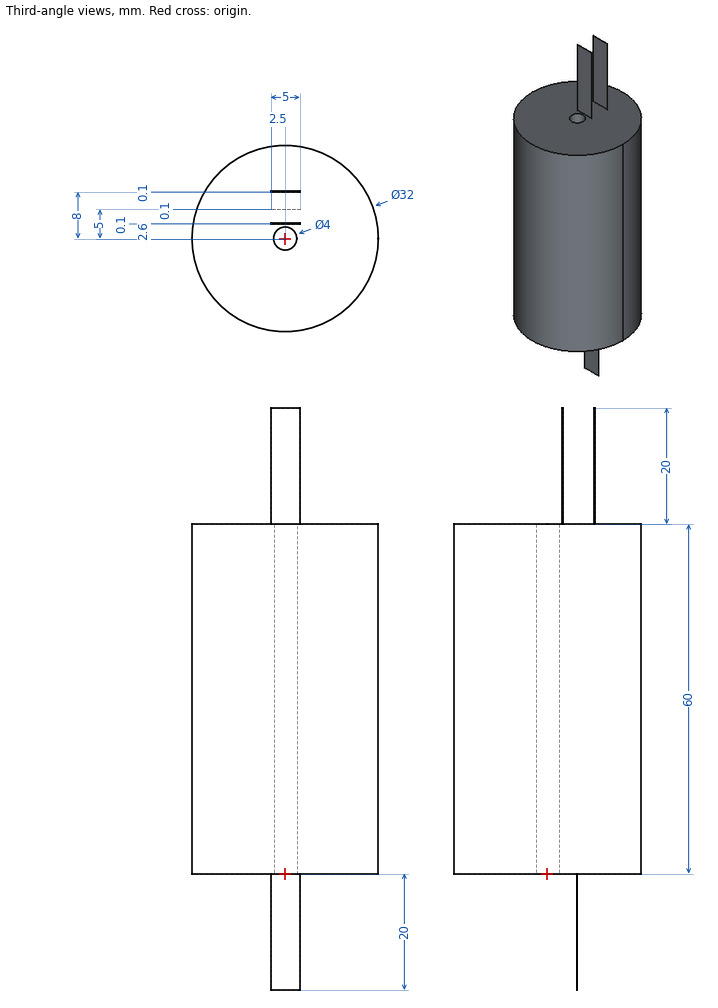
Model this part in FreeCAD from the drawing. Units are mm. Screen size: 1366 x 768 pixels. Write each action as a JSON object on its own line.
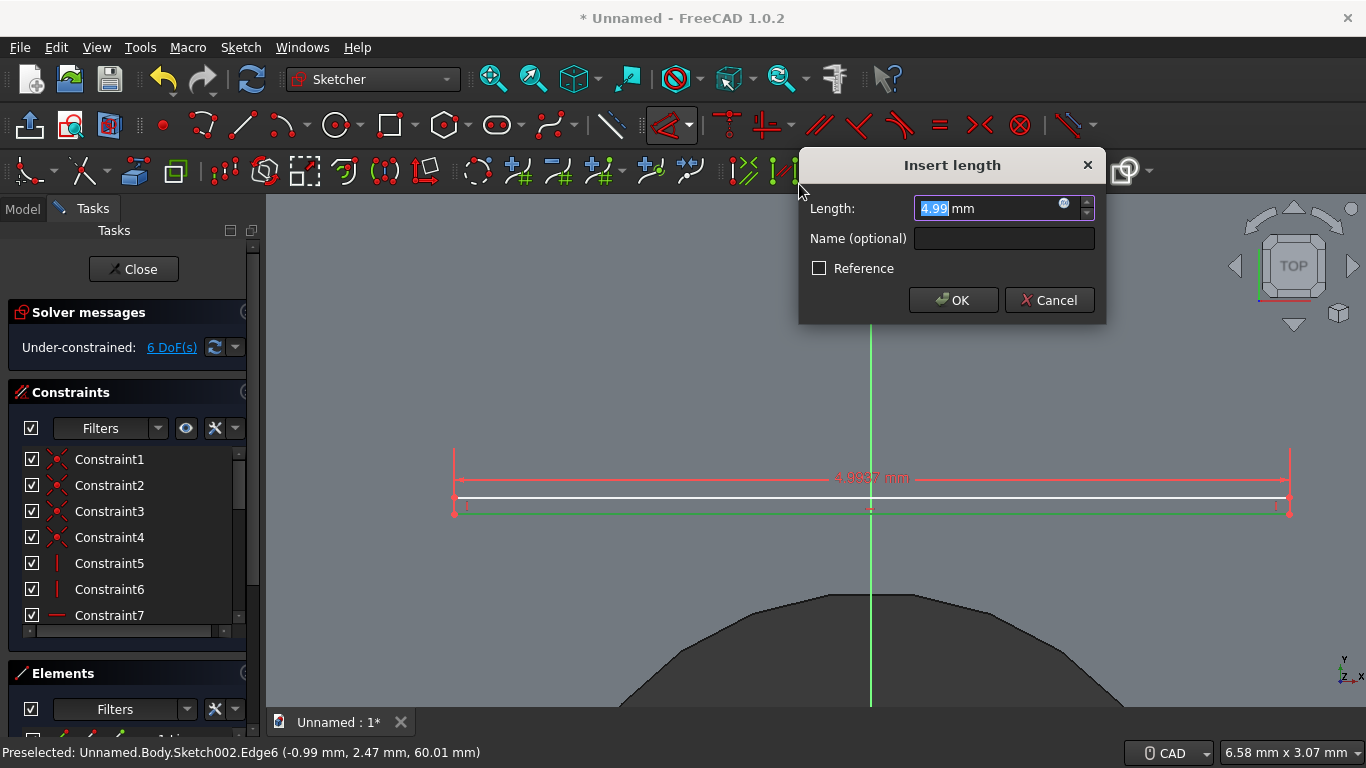
{"action": "type", "text": "5"}
{"action": "key", "text": "Return"}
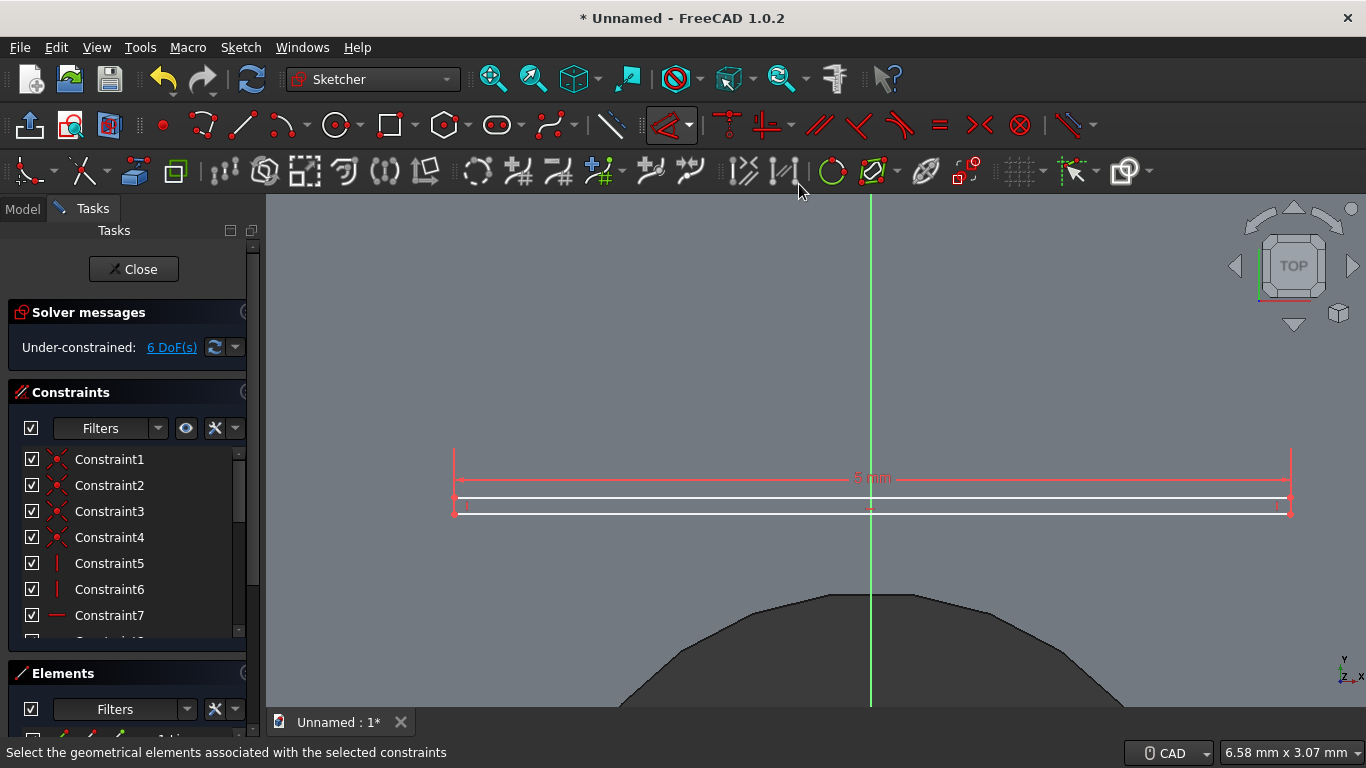
{"action": "scroll", "coordinate": [707, 516], "scroll_direction": "down", "scroll_amount": 7}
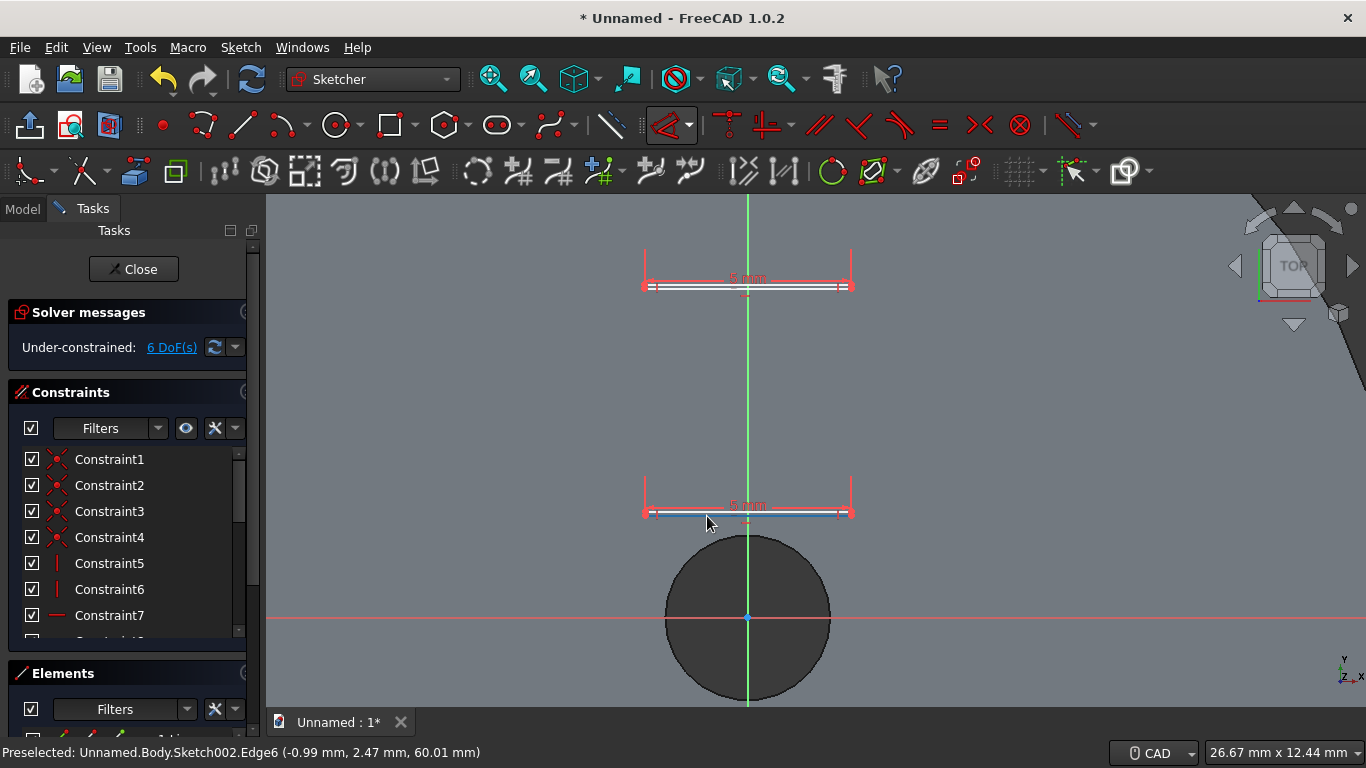
{"action": "scroll", "coordinate": [645, 289], "scroll_direction": "up", "scroll_amount": 6}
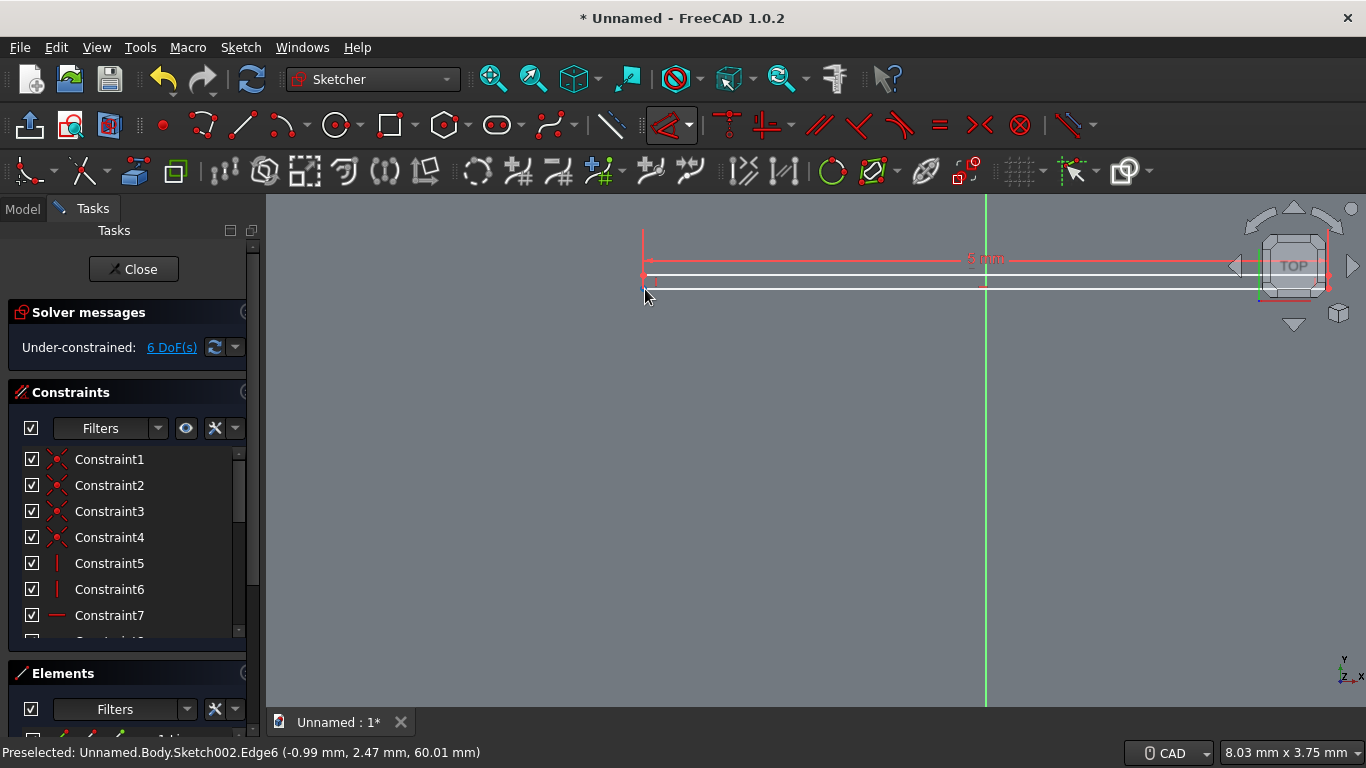
{"action": "left_click", "coordinate": [643, 289]}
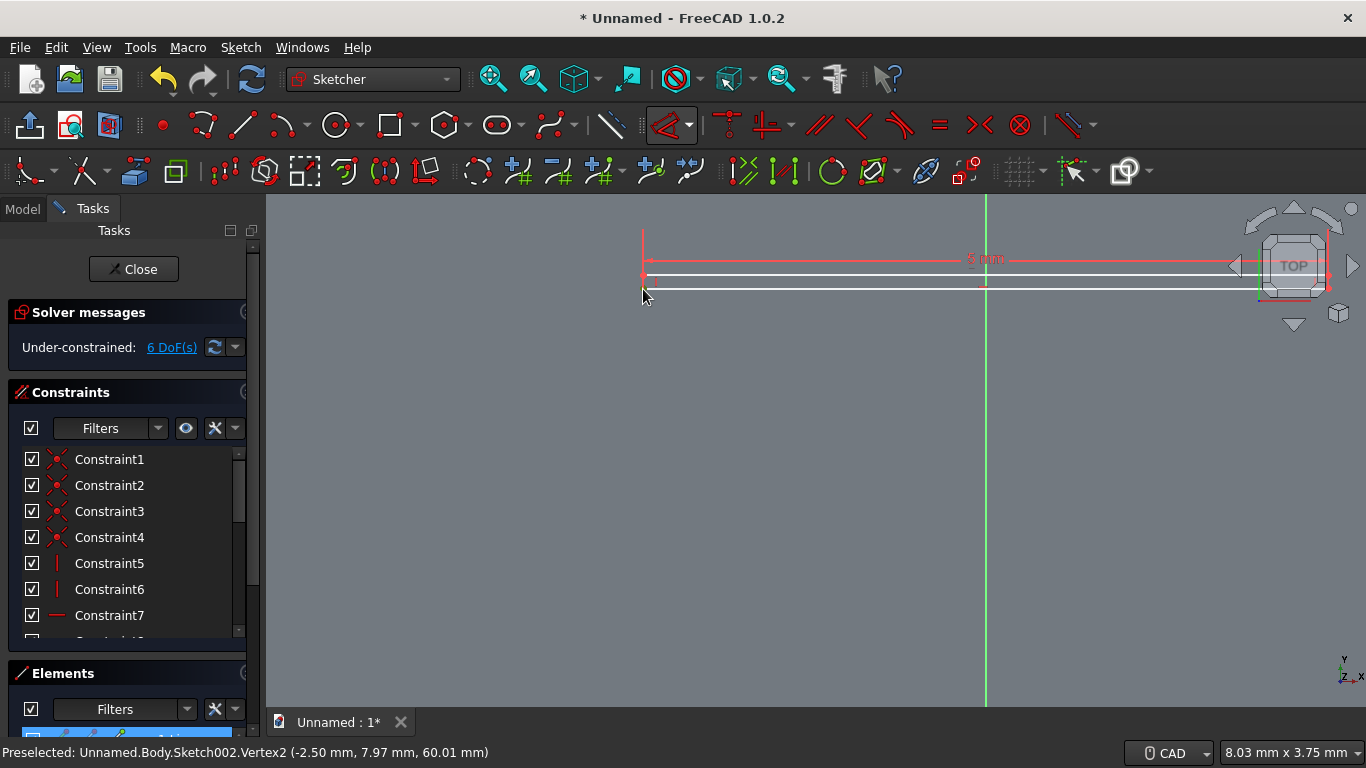
{"action": "left_click", "coordinate": [692, 126]}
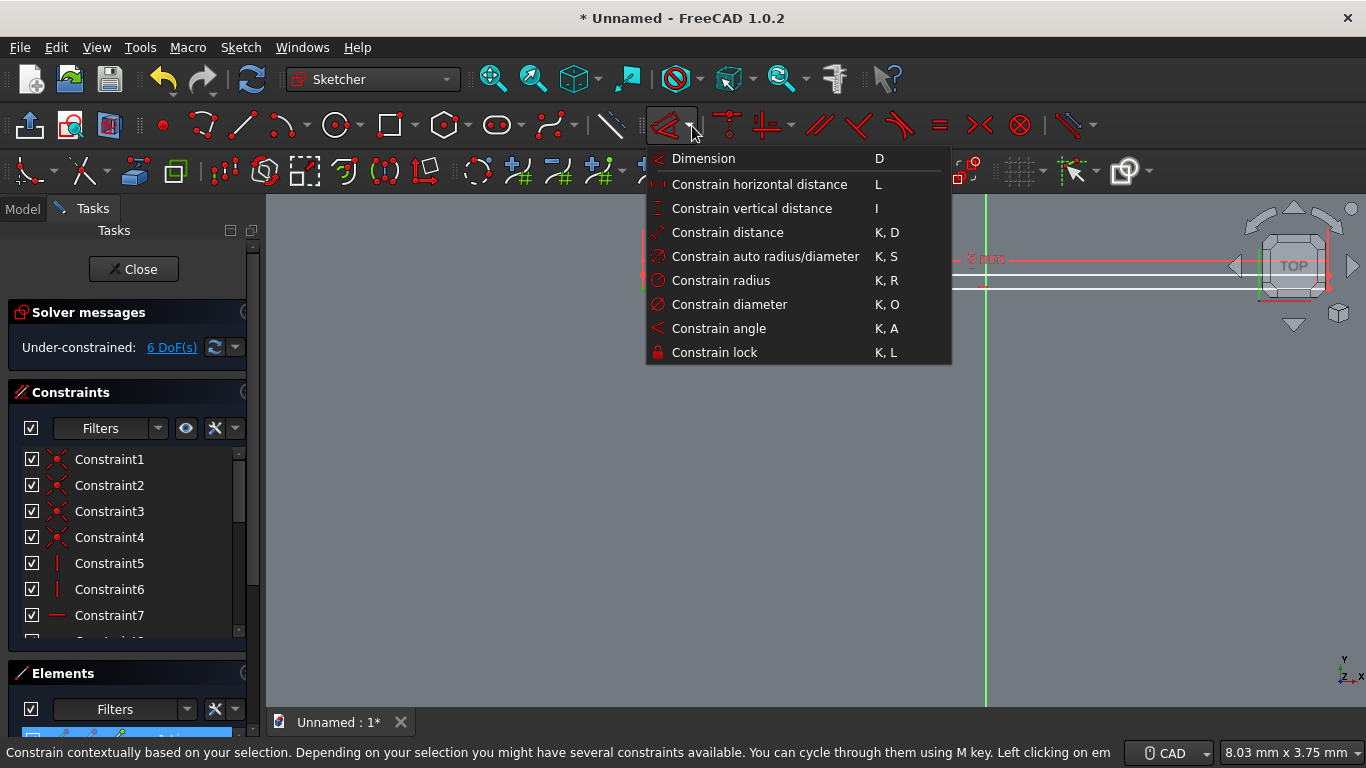
{"action": "left_click", "coordinate": [799, 208]}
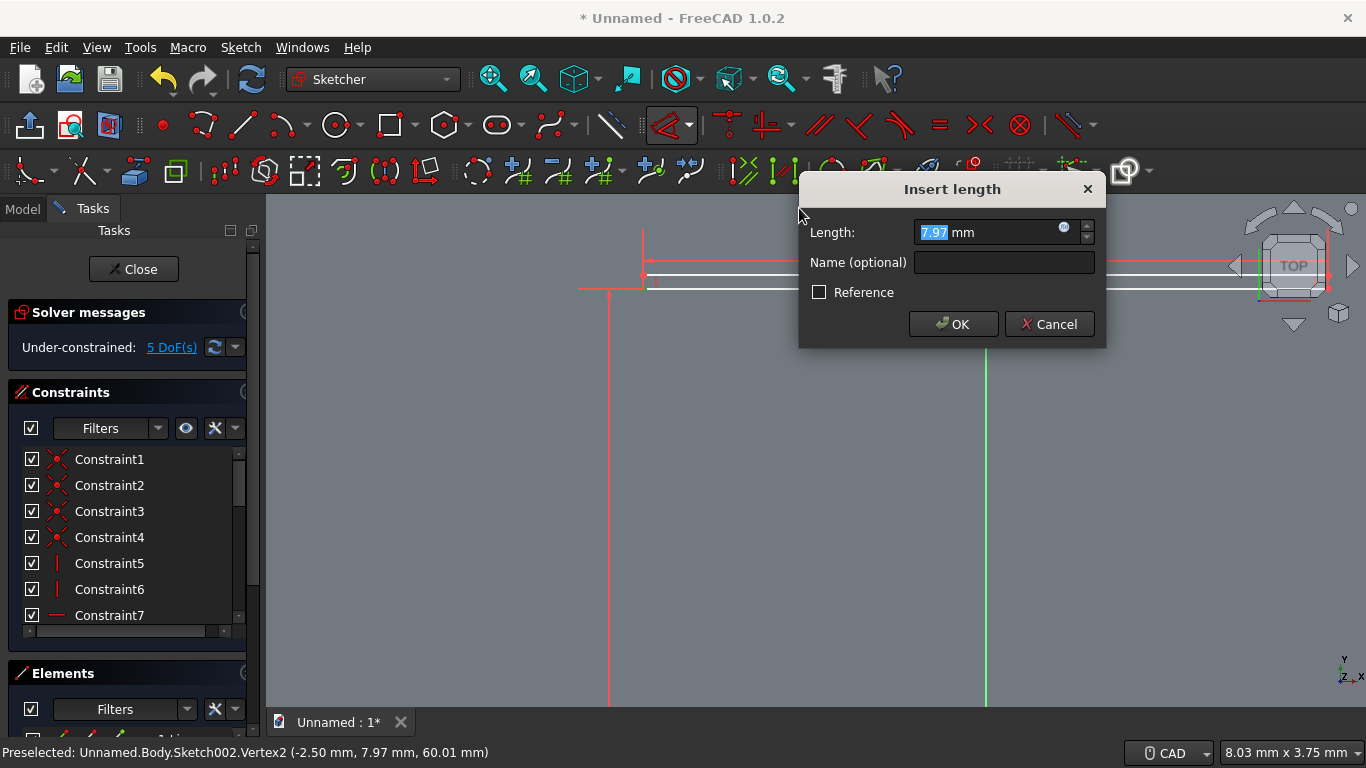
{"action": "type", "text": "8"}
{"action": "key", "text": "Return"}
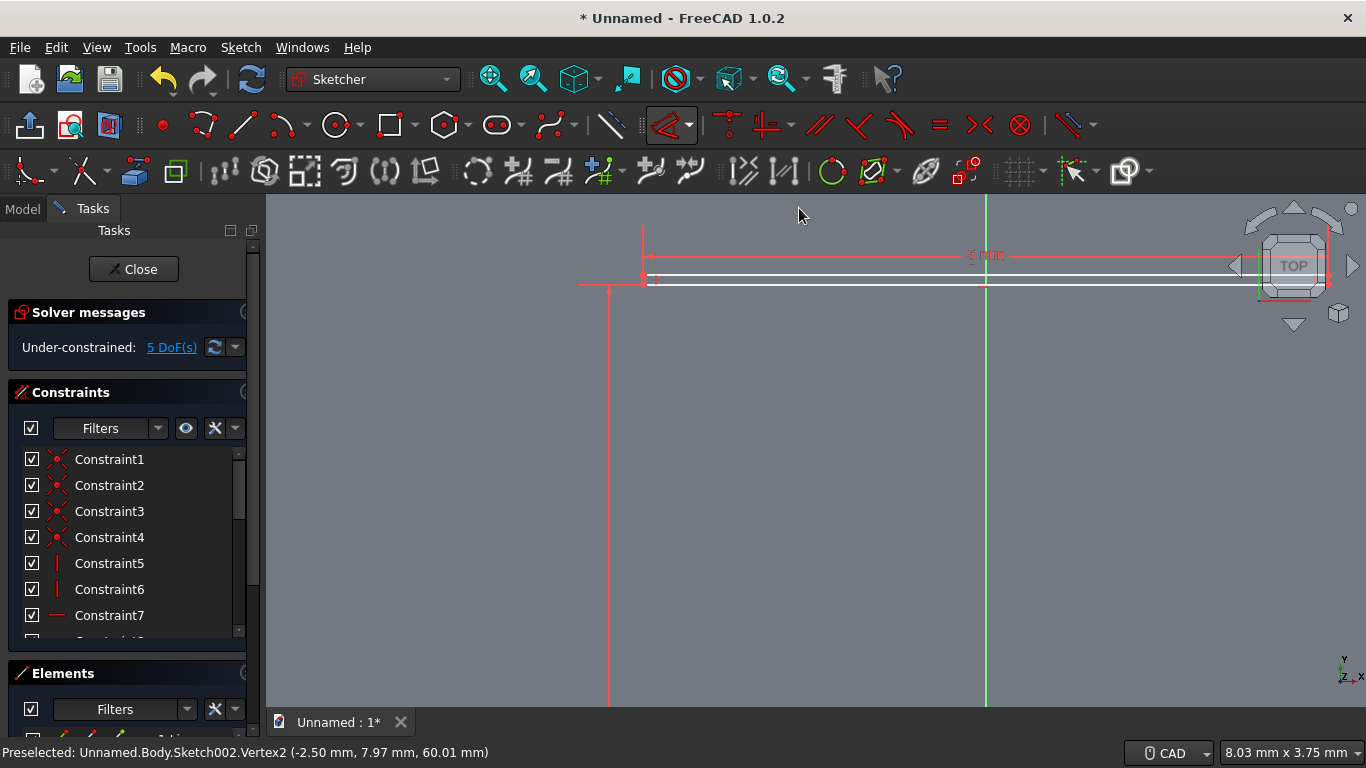
{"action": "scroll", "coordinate": [643, 280], "scroll_direction": "up", "scroll_amount": 6}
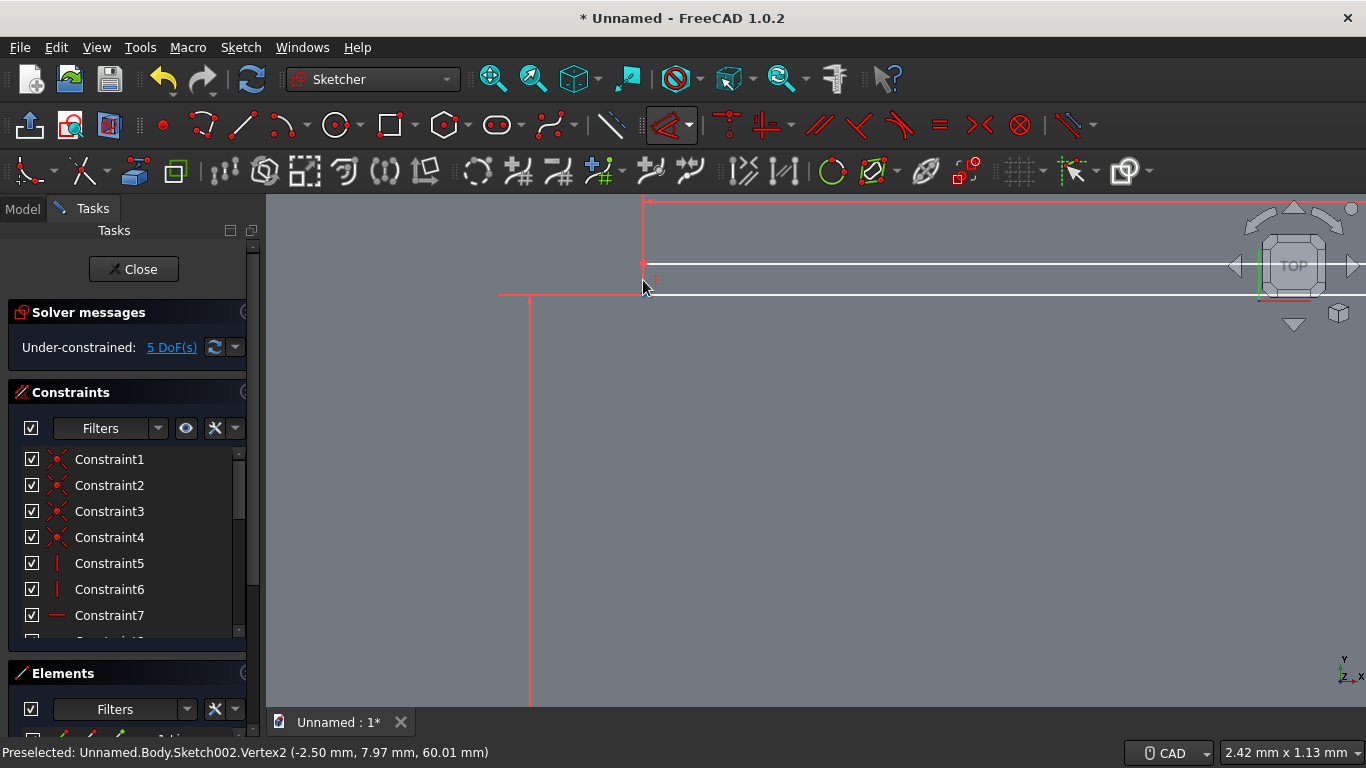
{"action": "left_click", "coordinate": [643, 279]}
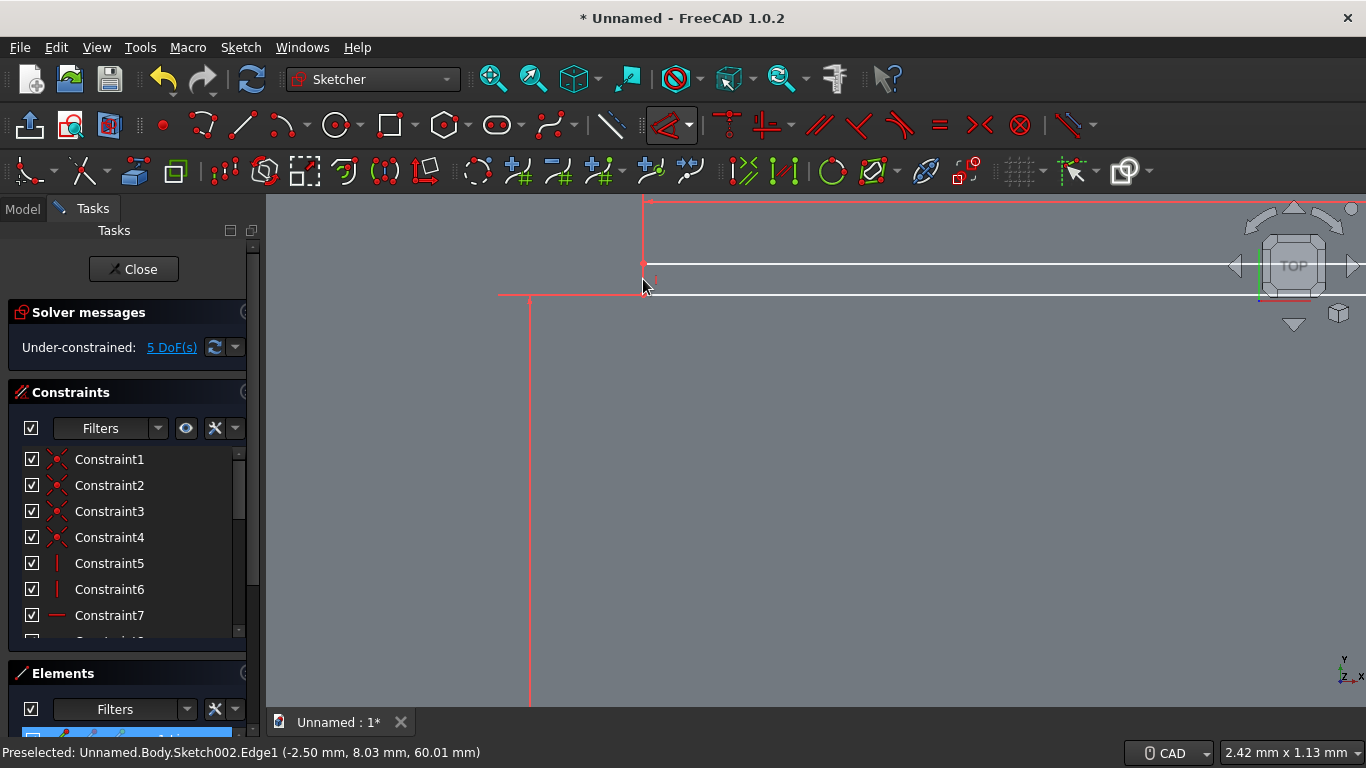
{"action": "left_click", "coordinate": [692, 126]}